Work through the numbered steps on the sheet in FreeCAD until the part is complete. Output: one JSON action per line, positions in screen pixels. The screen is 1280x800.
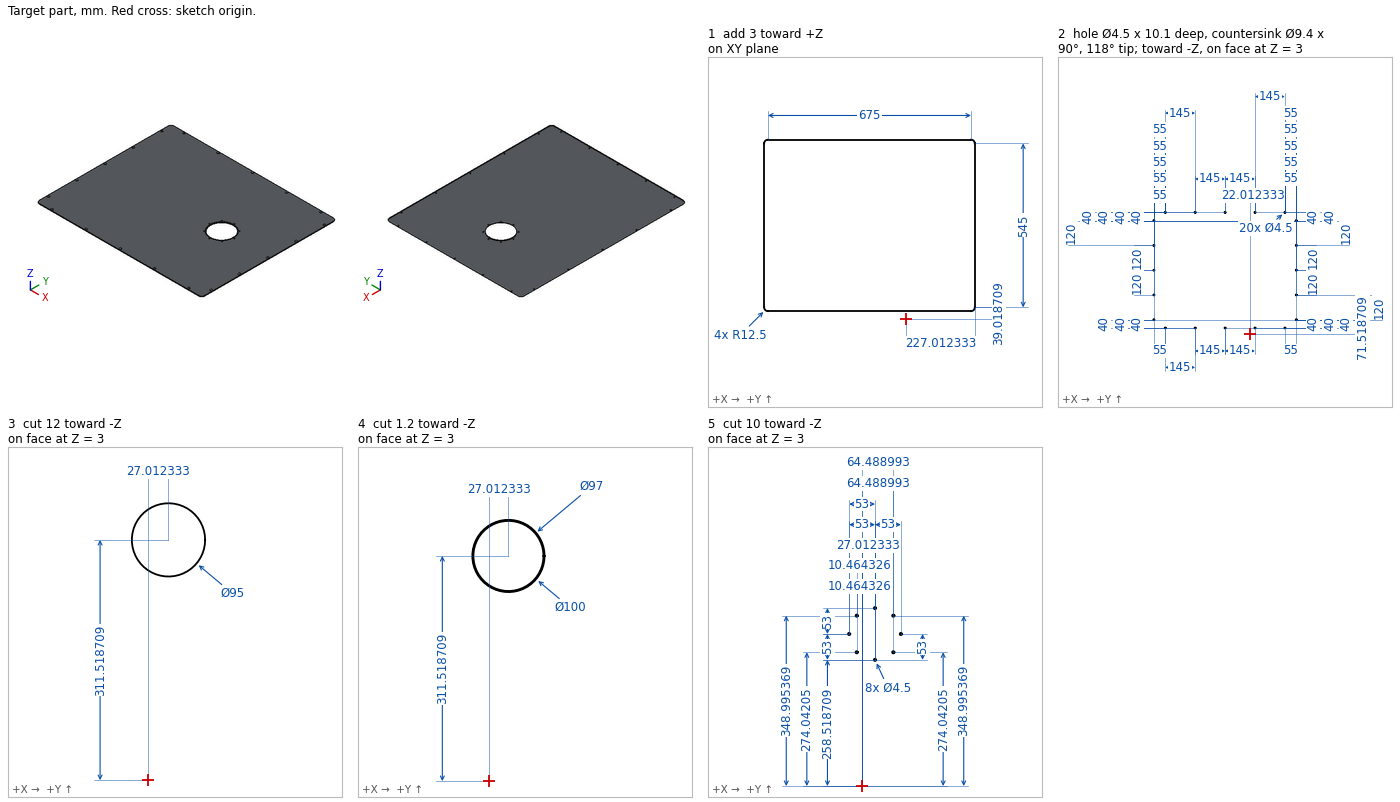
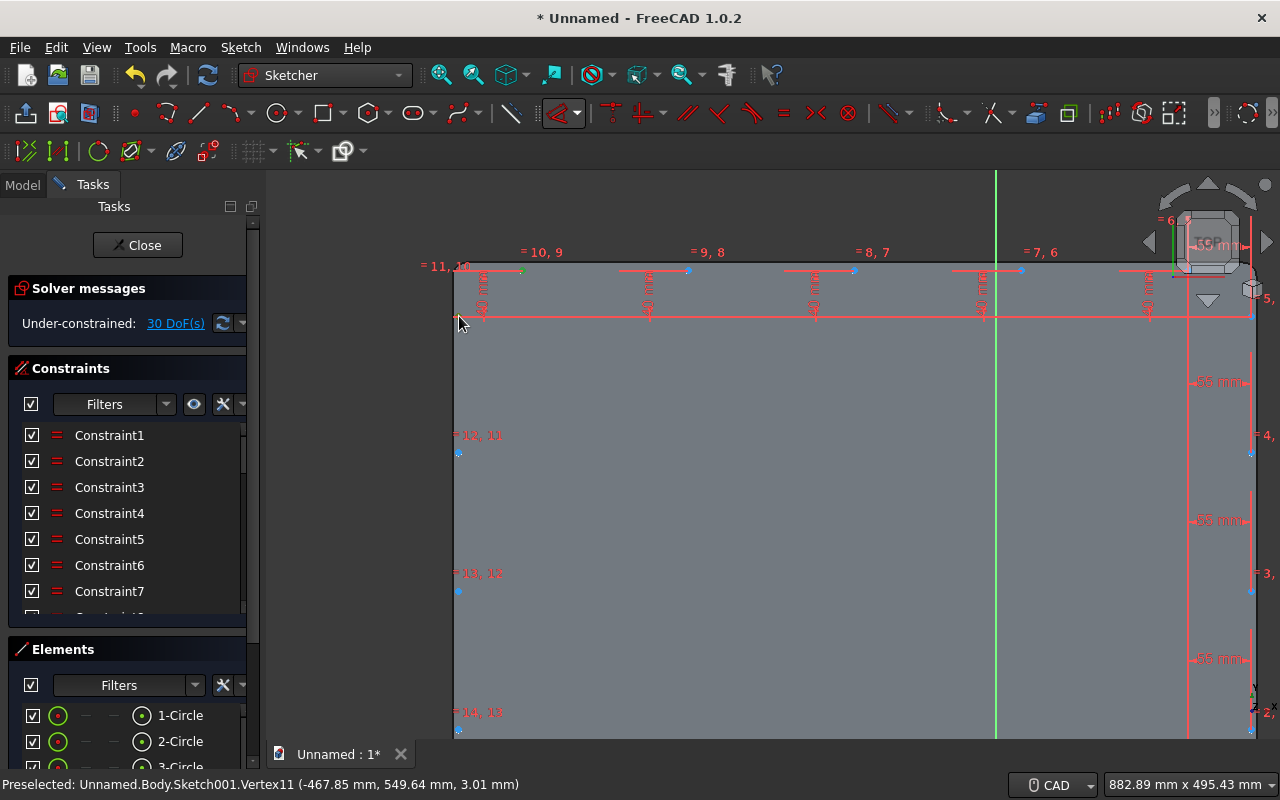
{"action": "left_click", "coordinate": [580, 114]}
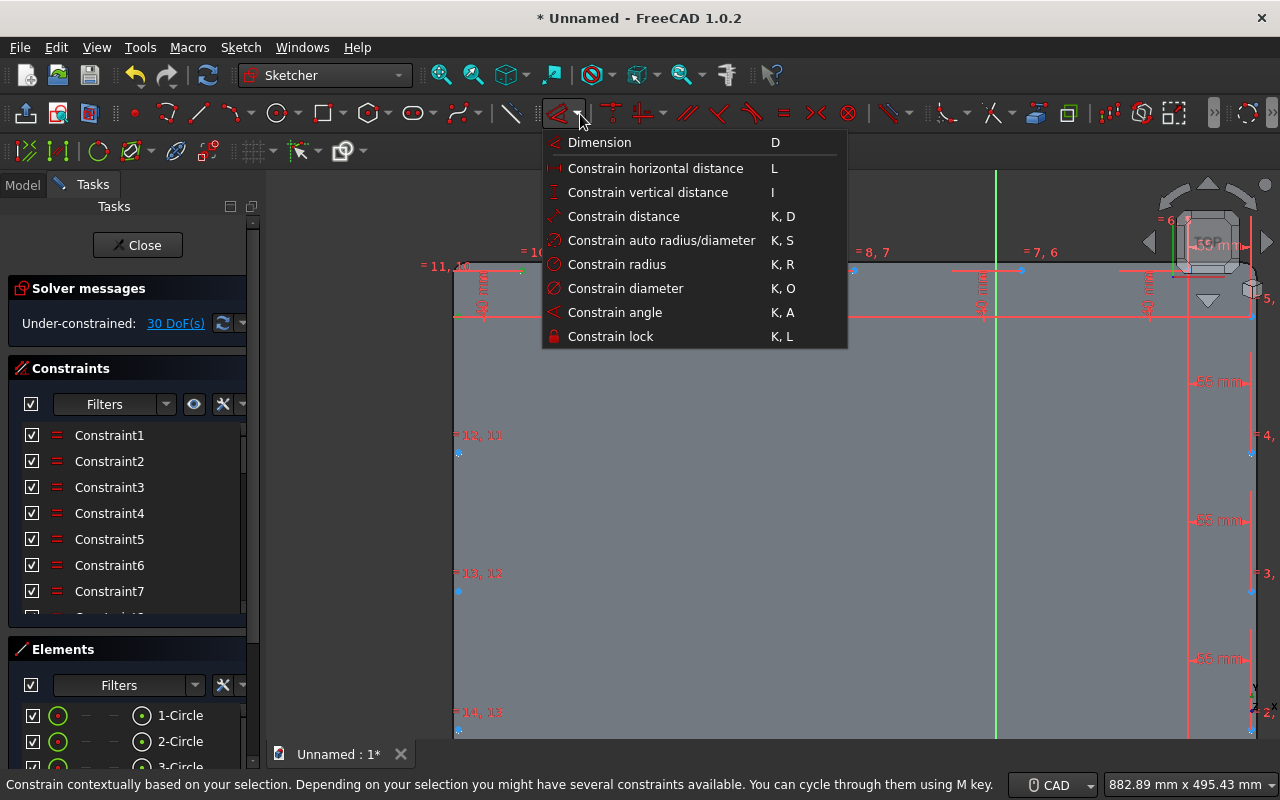
{"action": "left_click", "coordinate": [695, 168]}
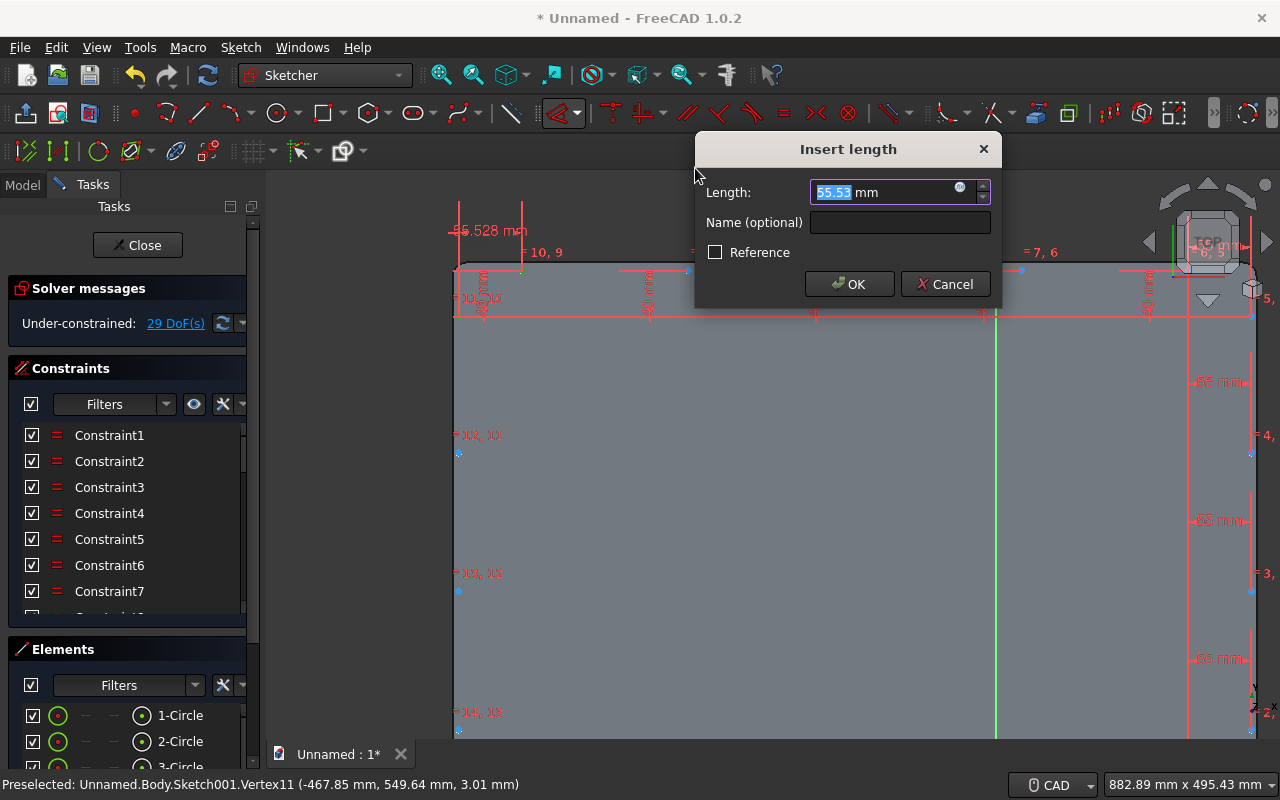
{"action": "type", "text": "55"}
{"action": "key", "text": "Return"}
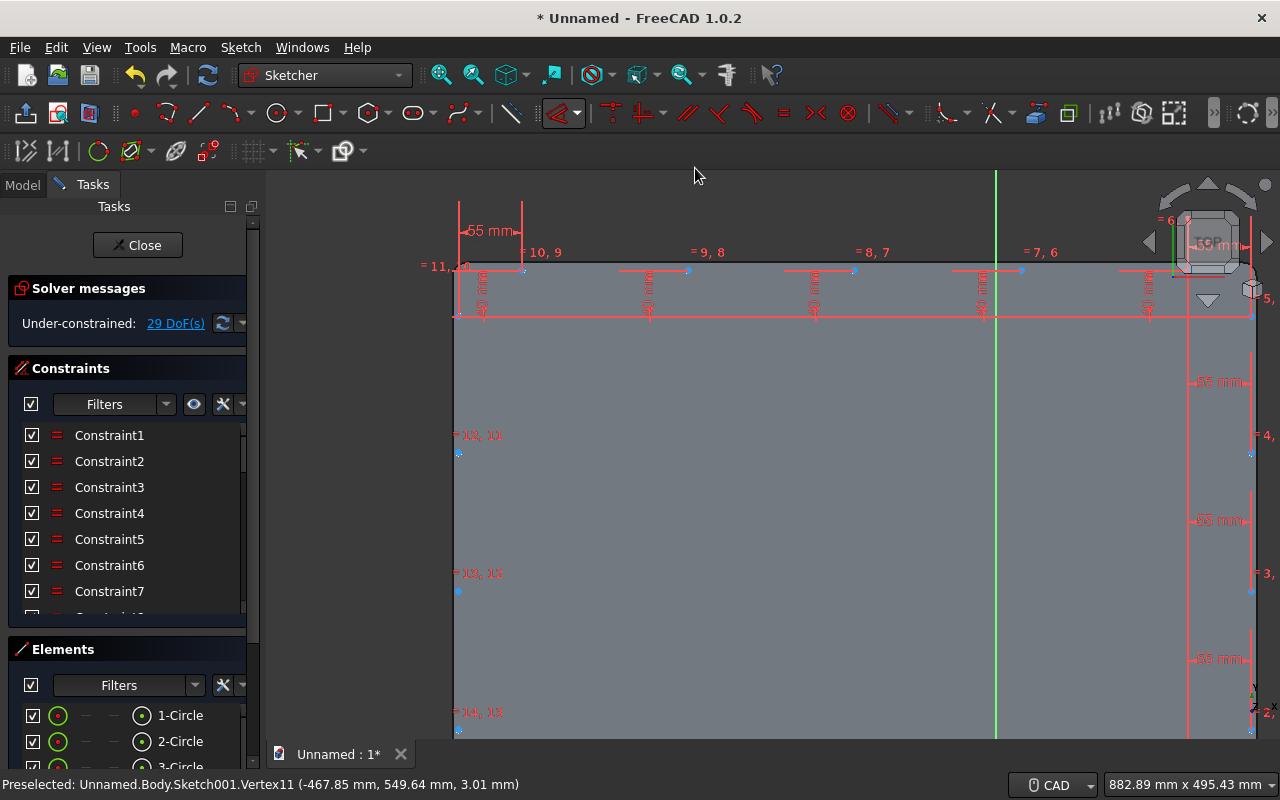
{"action": "left_click", "coordinate": [522, 271]}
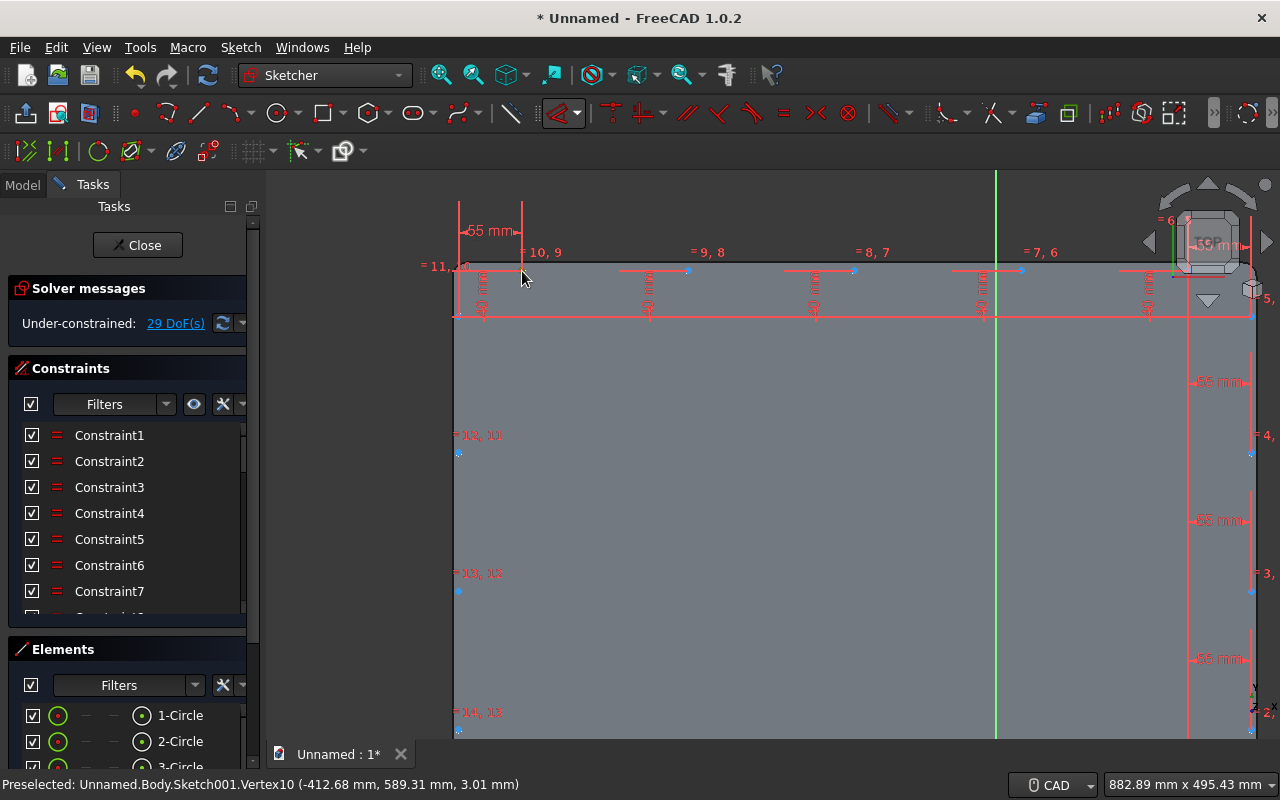
{"action": "left_click", "coordinate": [459, 316]}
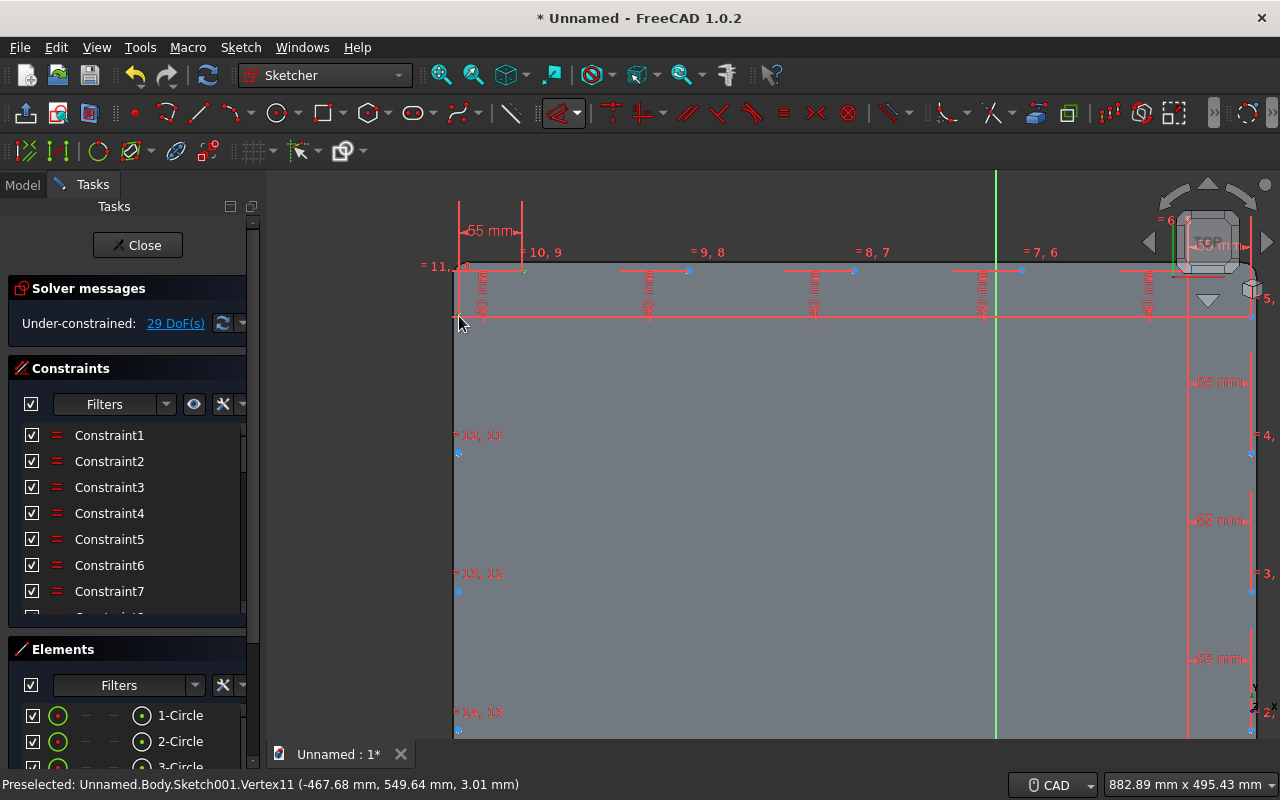
{"action": "key", "text": "i"}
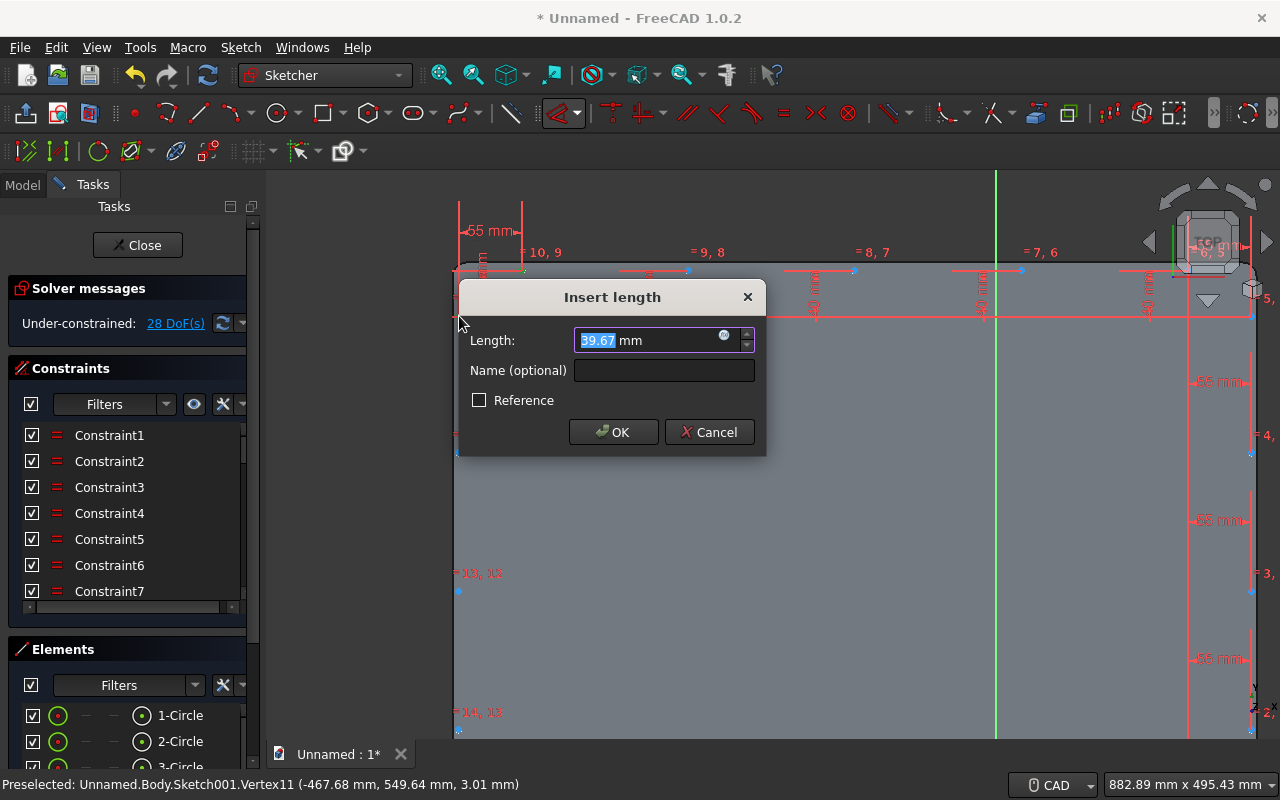
{"action": "type", "text": "40"}
{"action": "key", "text": "Return"}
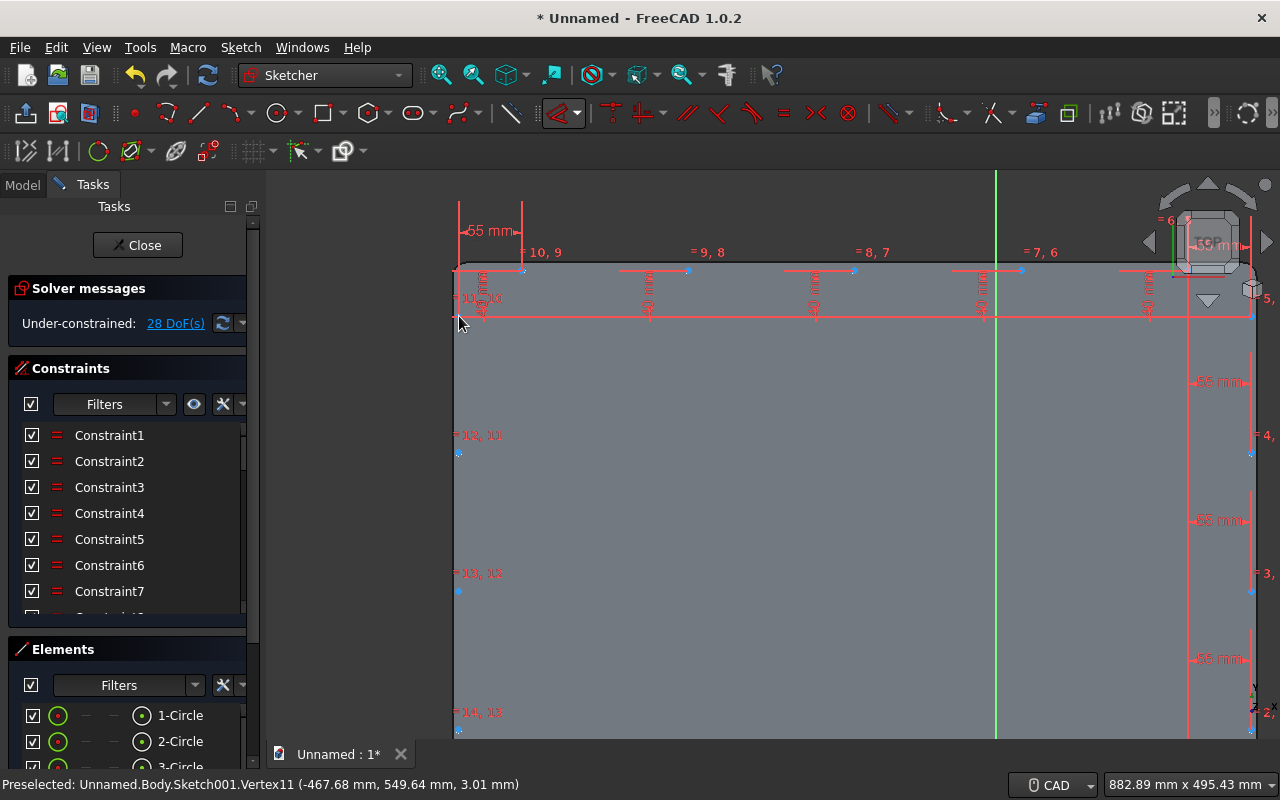
{"action": "left_click", "coordinate": [522, 271]}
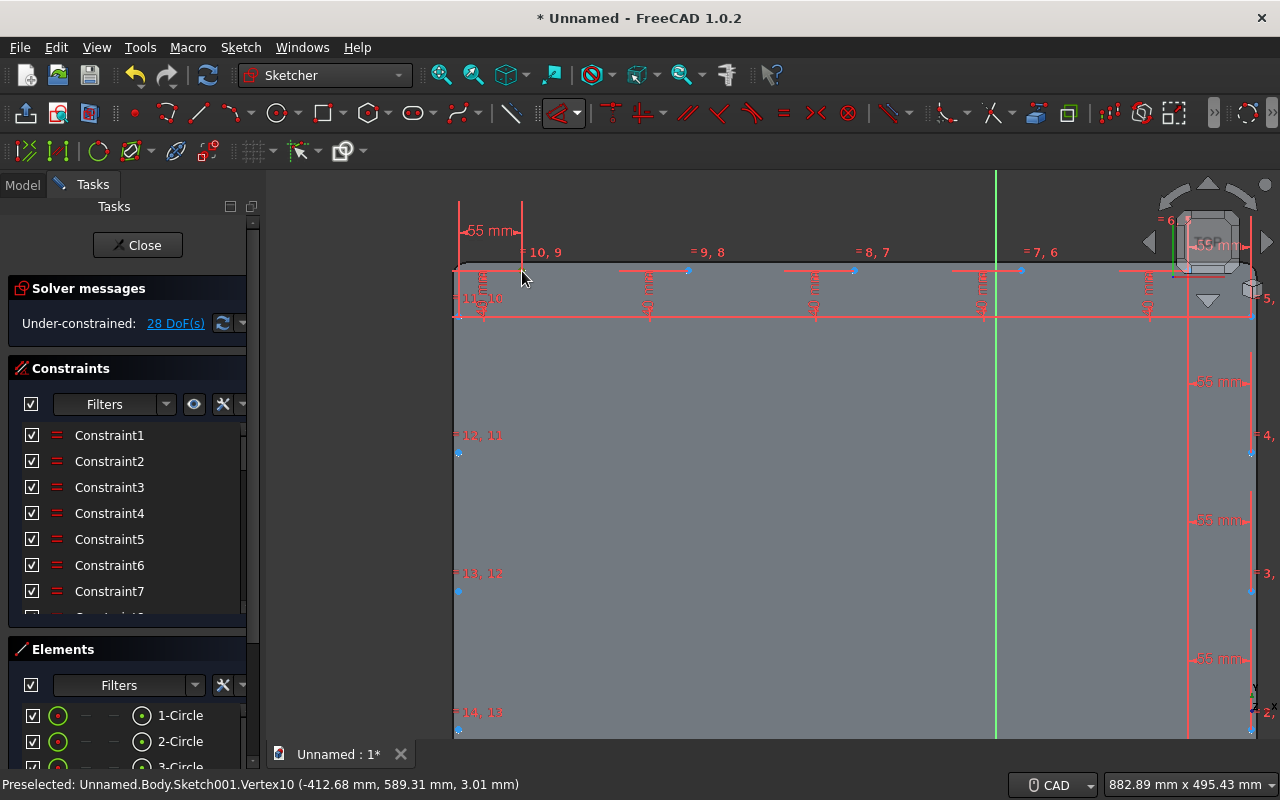
{"action": "left_click", "coordinate": [459, 453]}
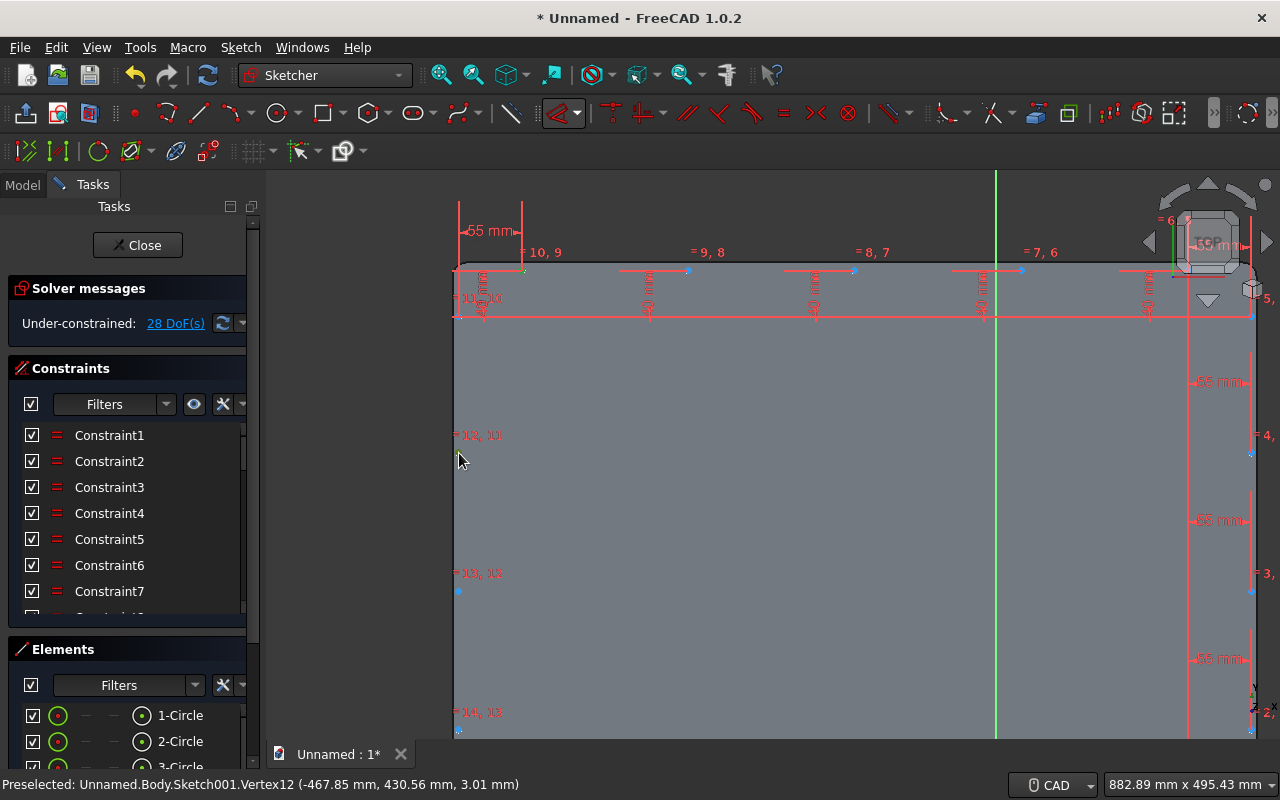
{"action": "key", "text": "l"}